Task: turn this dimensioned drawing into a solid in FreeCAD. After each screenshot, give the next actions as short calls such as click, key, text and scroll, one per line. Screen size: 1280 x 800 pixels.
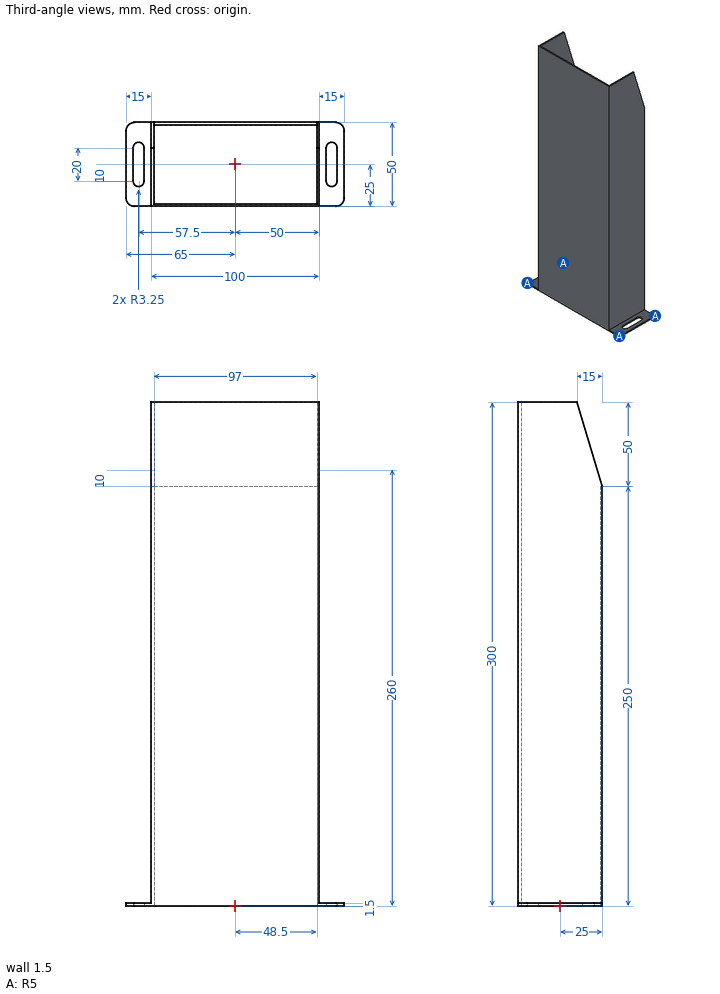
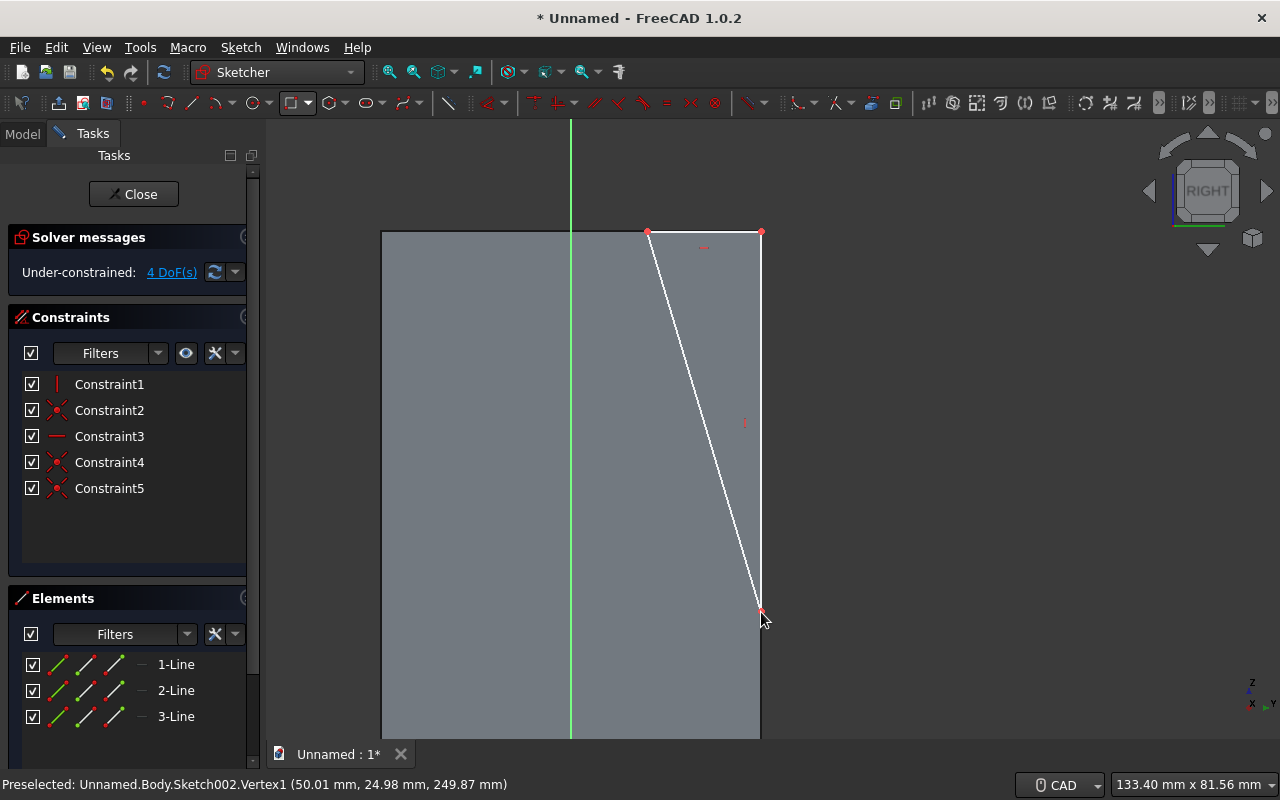
click(488, 104)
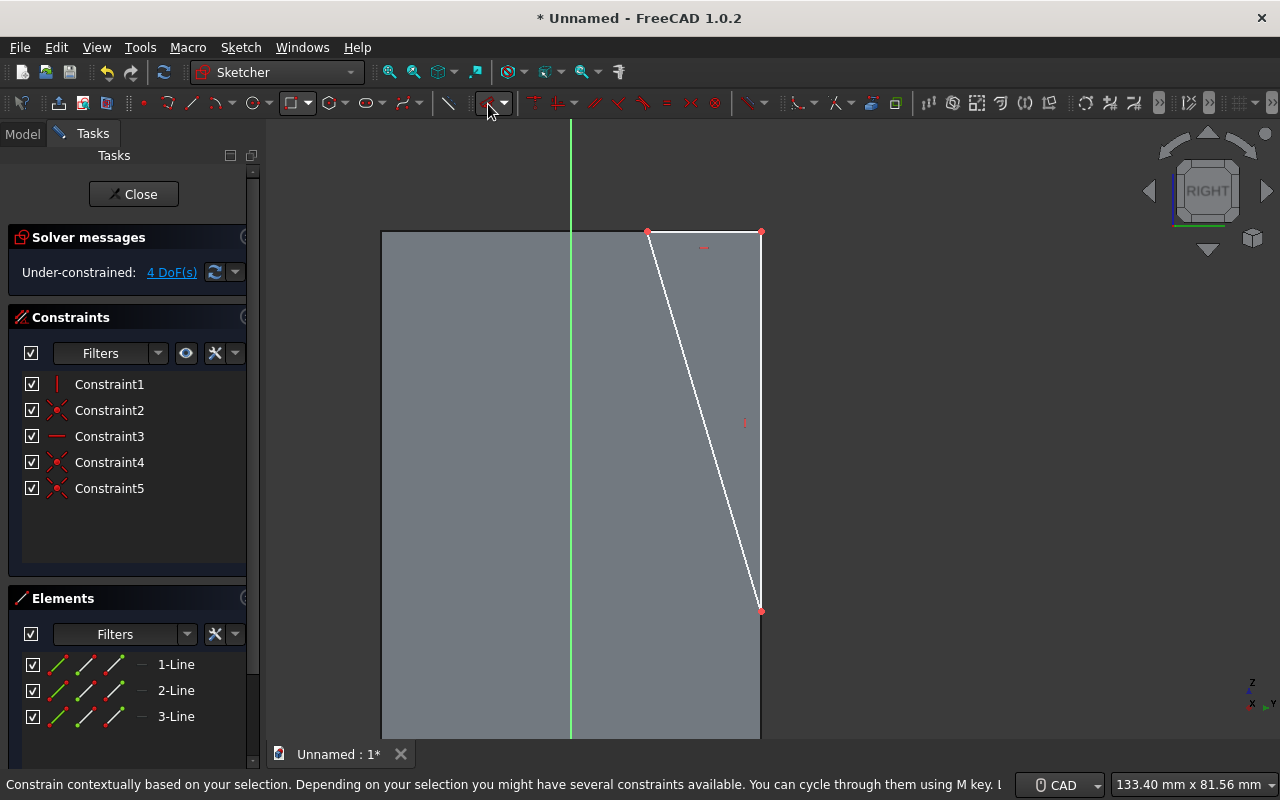
click(761, 498)
click(795, 422)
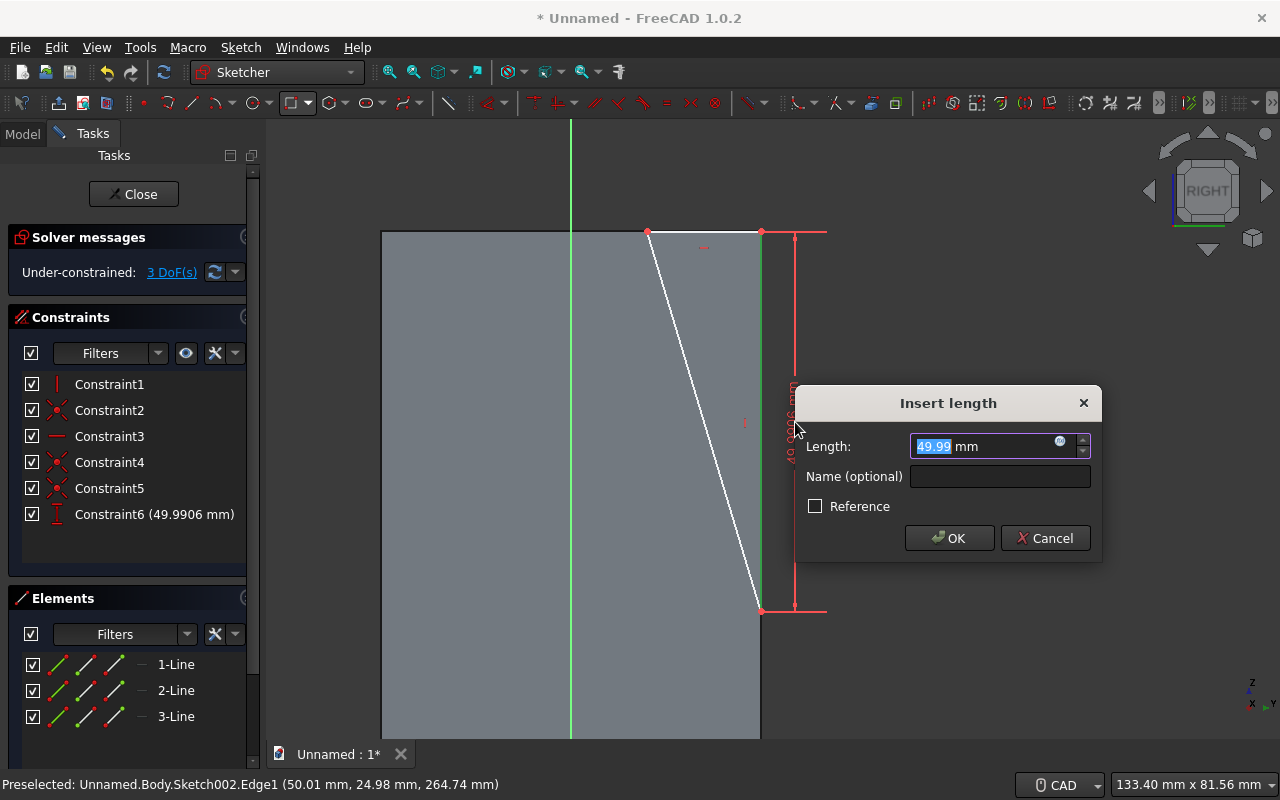
text(50)
key(Return)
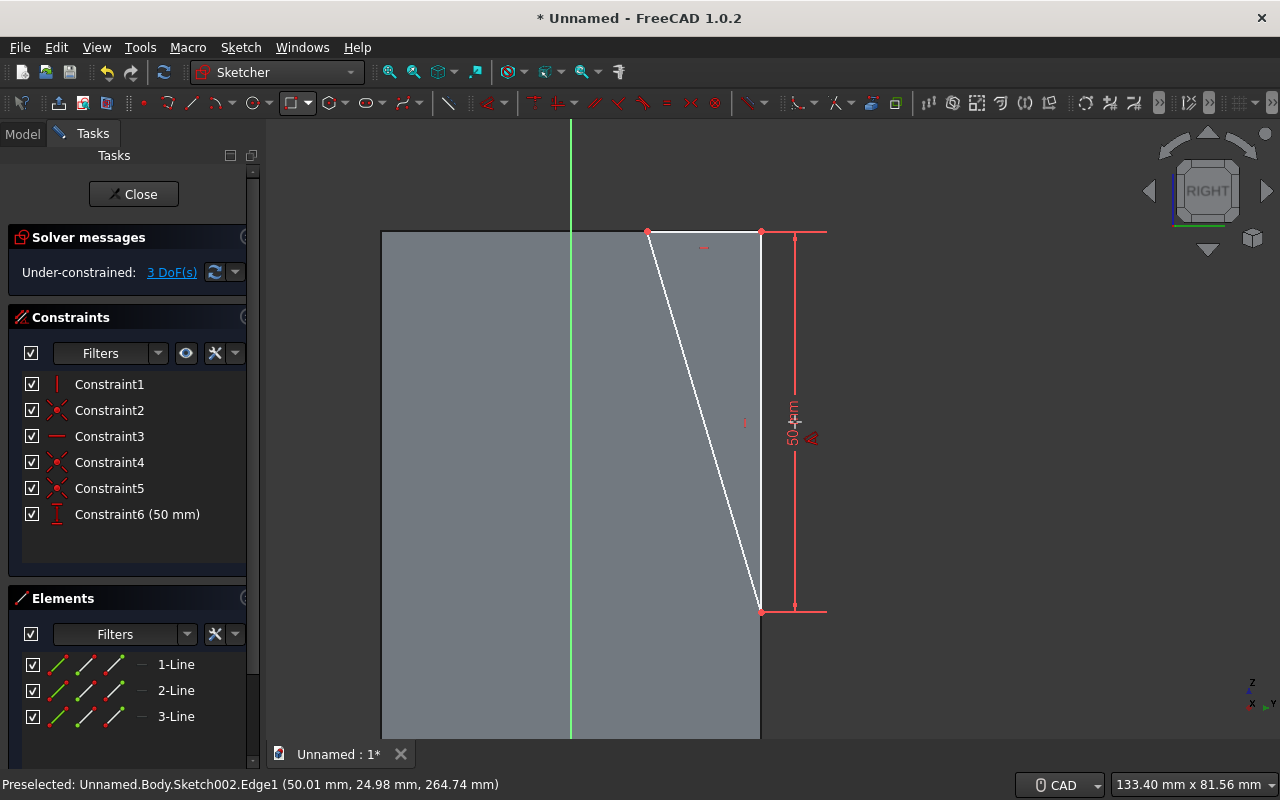
click(727, 232)
click(704, 198)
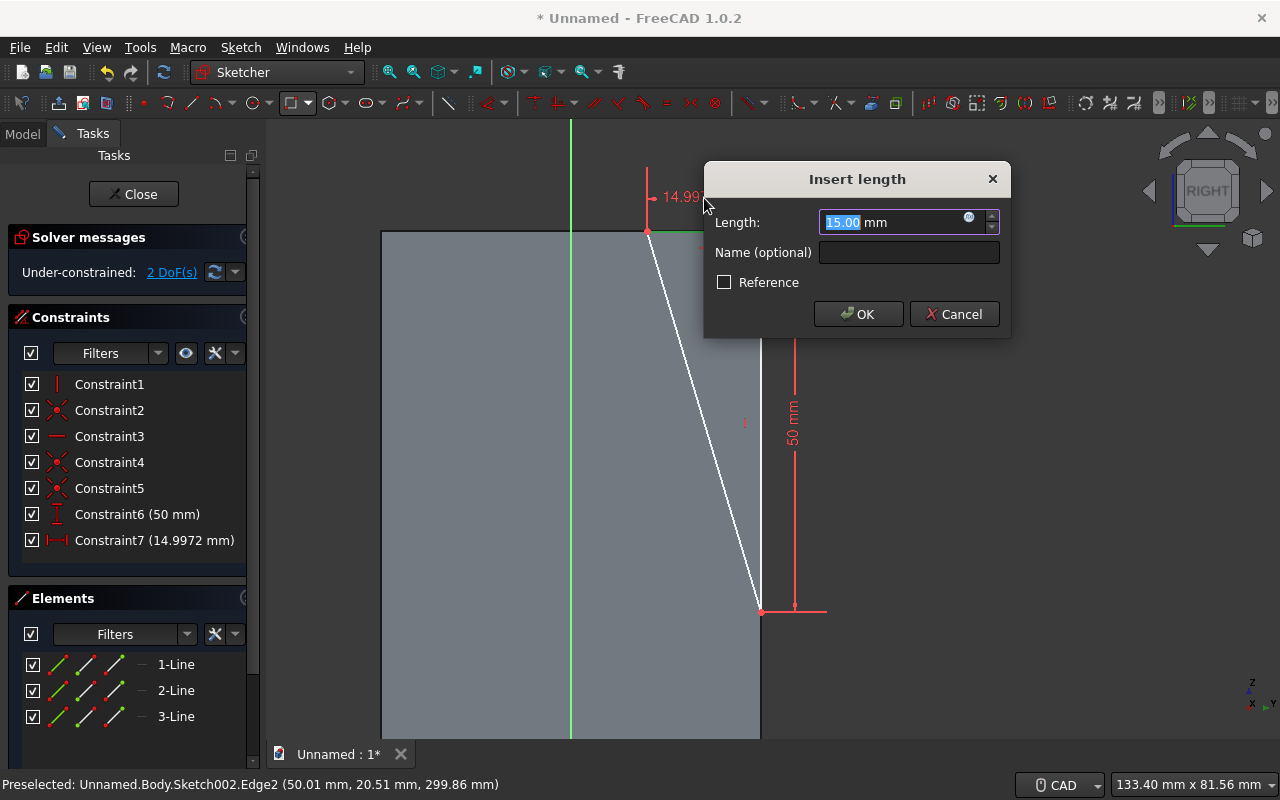
text(15)
key(Return)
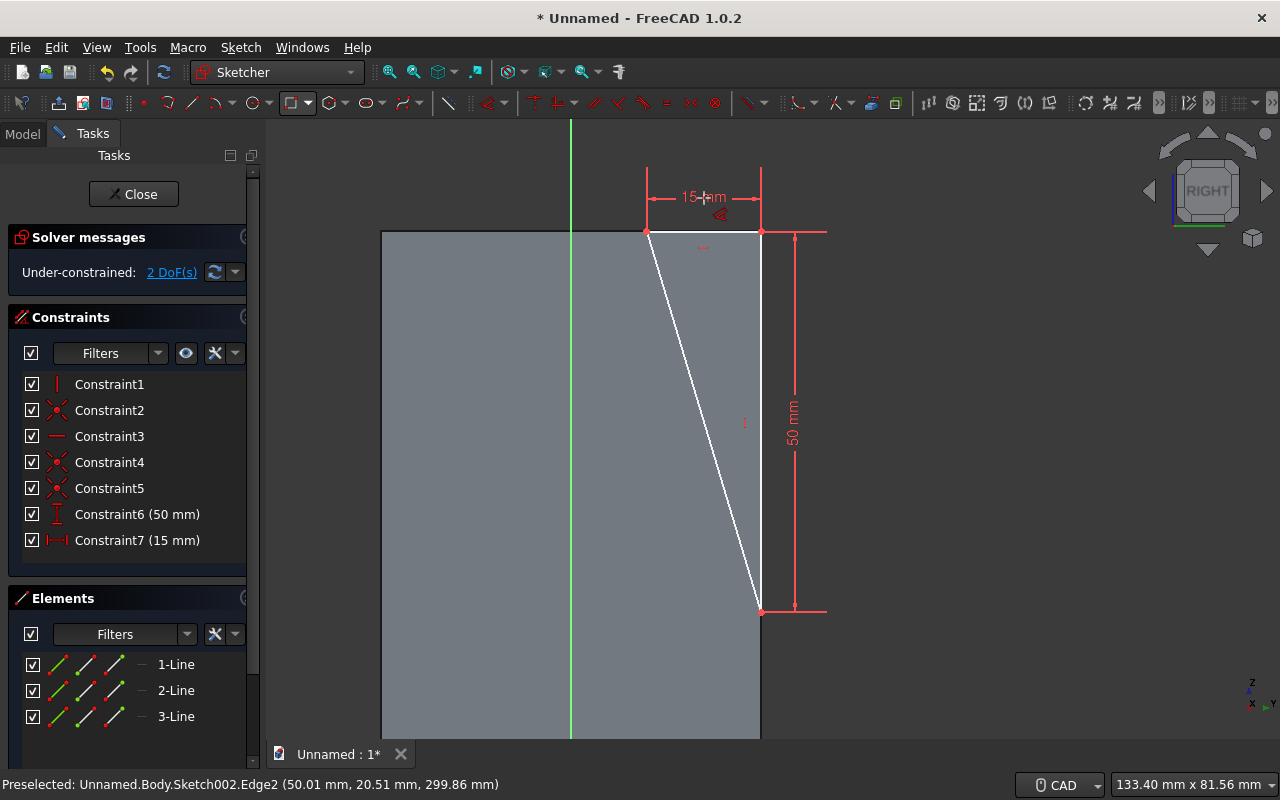
click(761, 612)
click(666, 578)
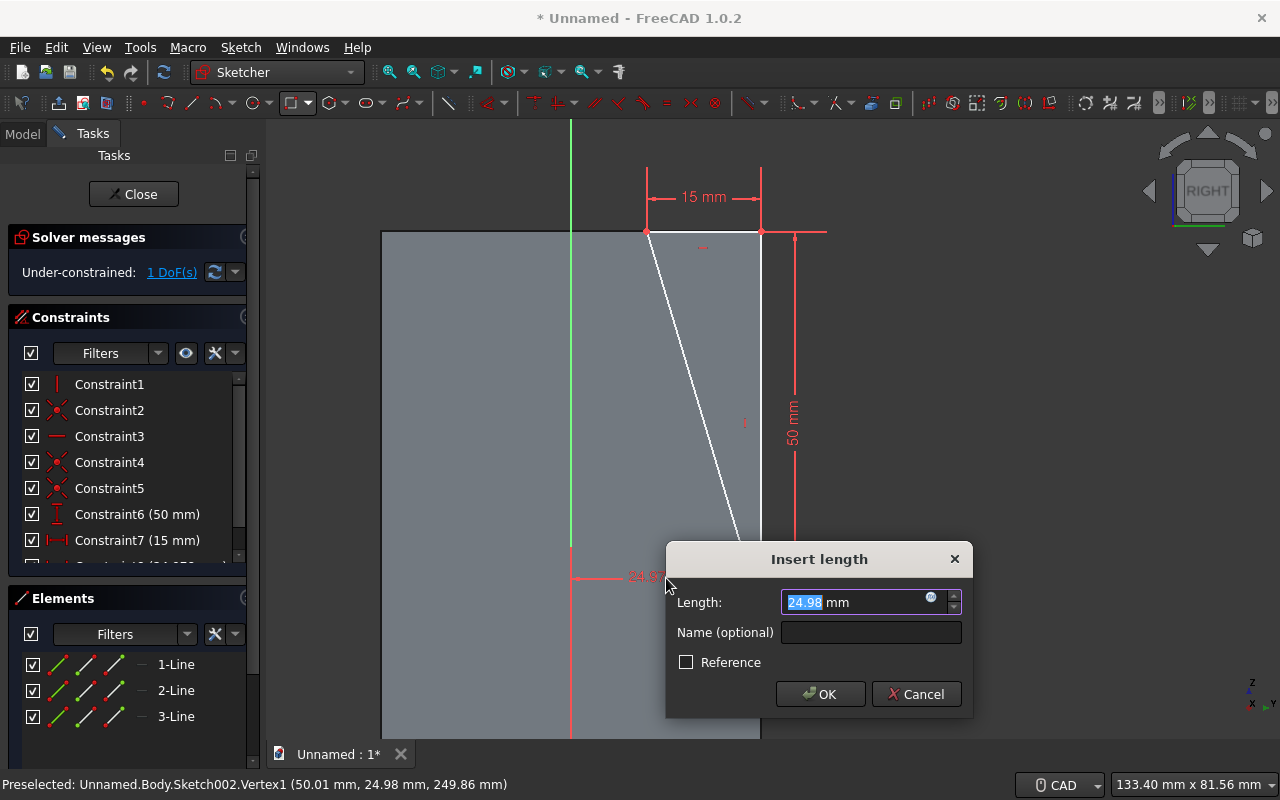
text(25)
key(Return)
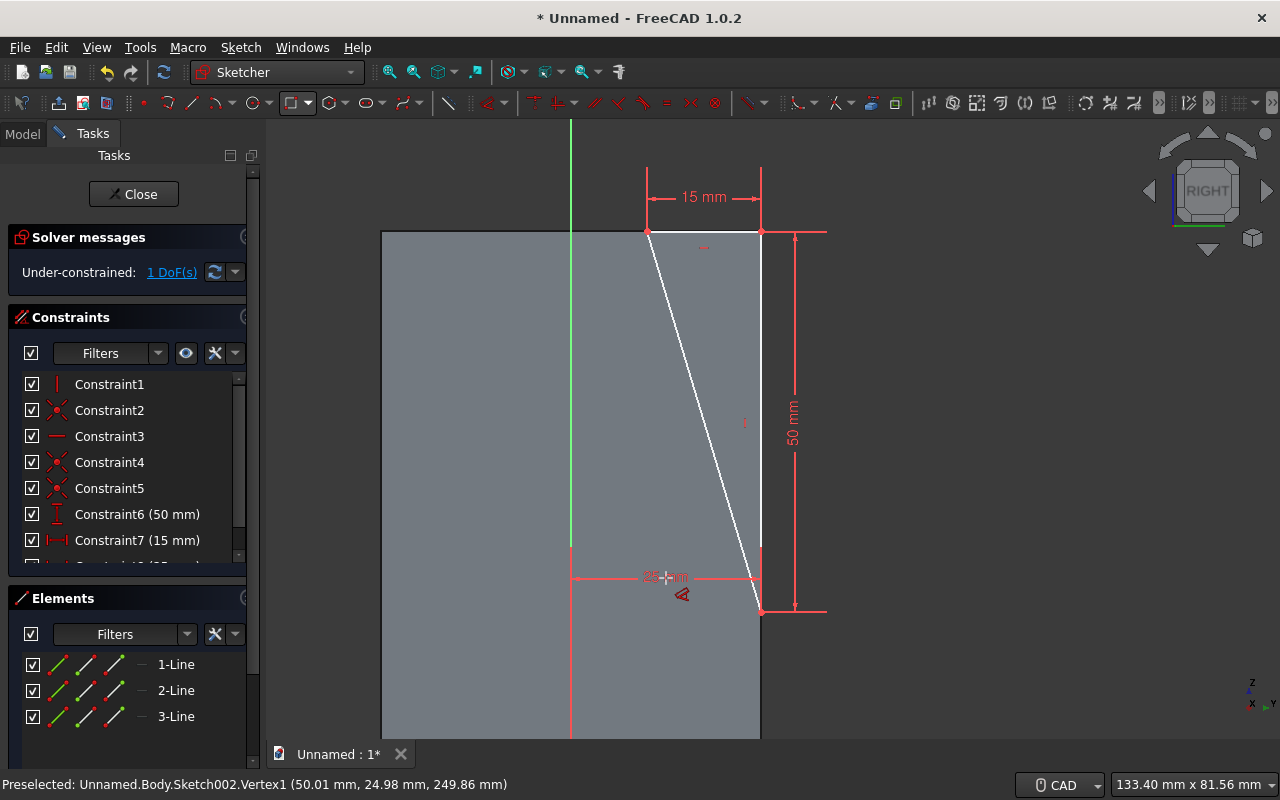
click(761, 612)
click(537, 662)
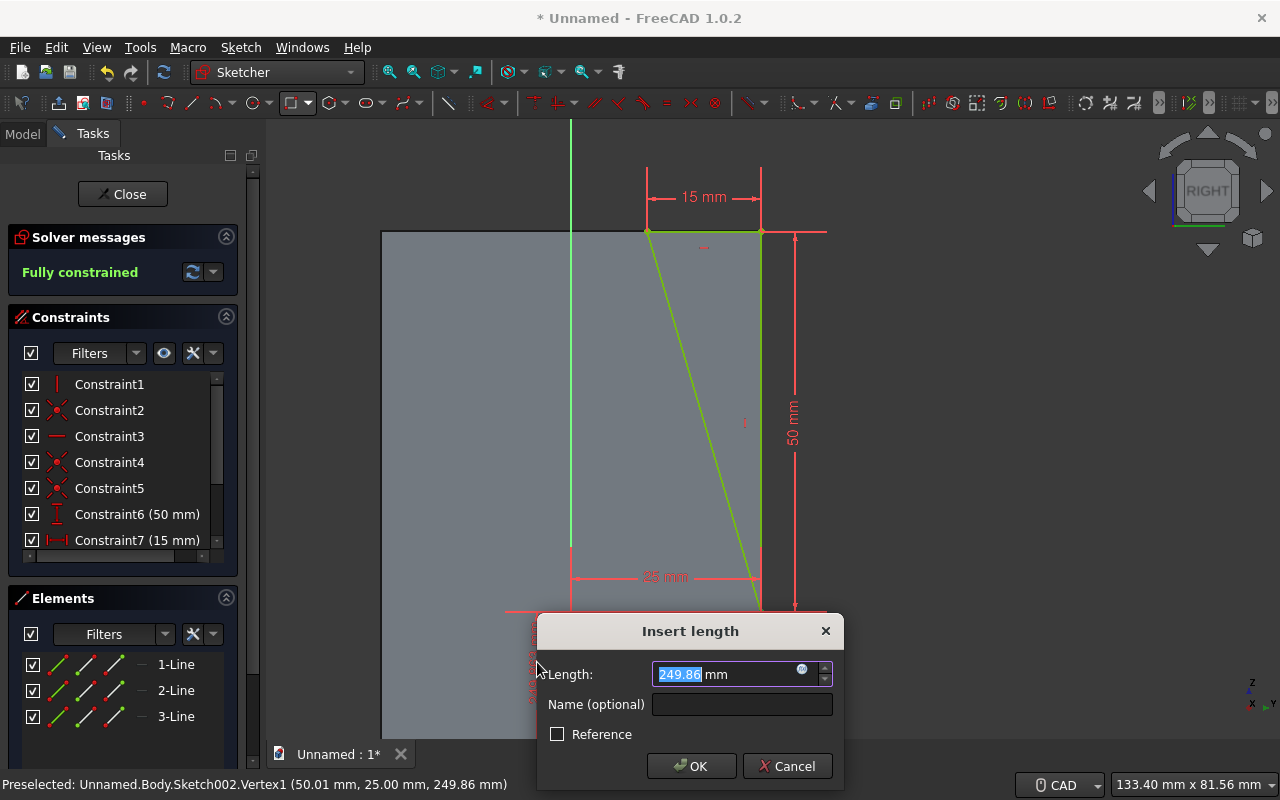
text(250)
key(Return)
key(Escape)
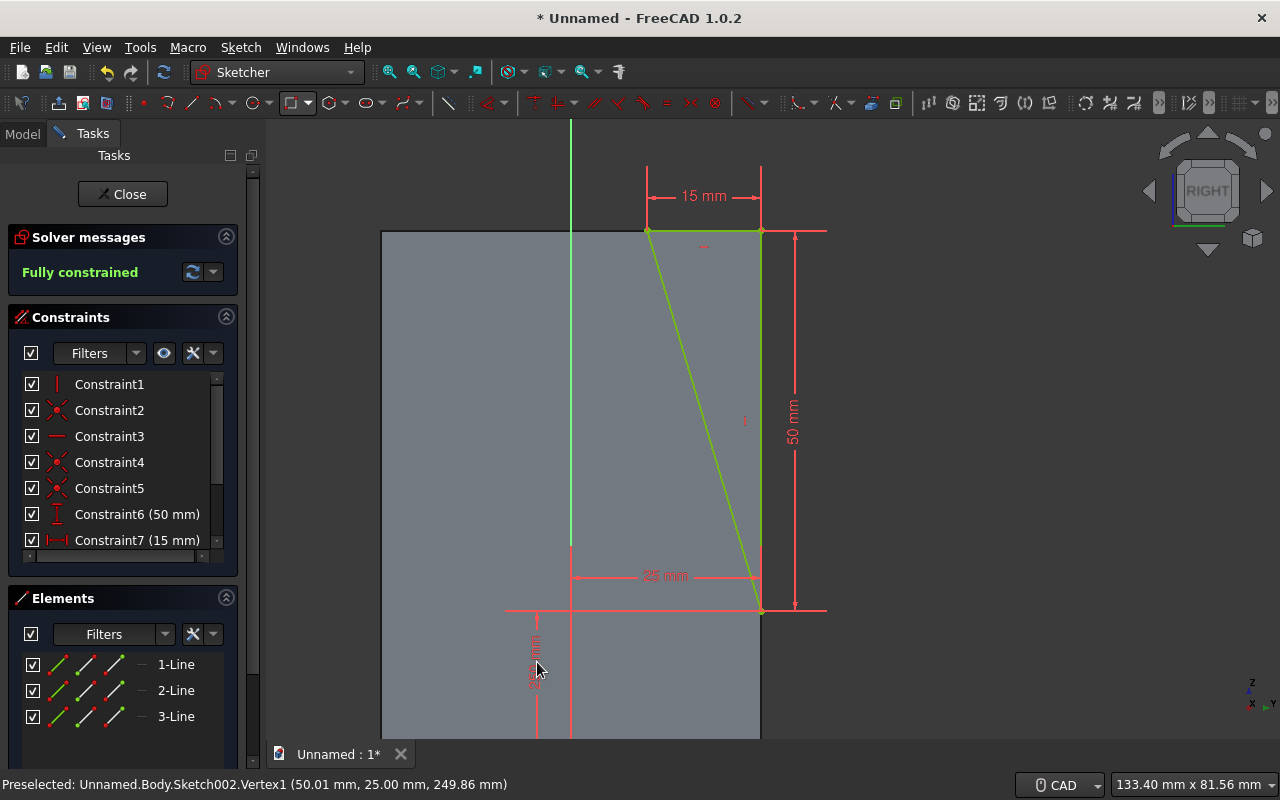
click(123, 194)